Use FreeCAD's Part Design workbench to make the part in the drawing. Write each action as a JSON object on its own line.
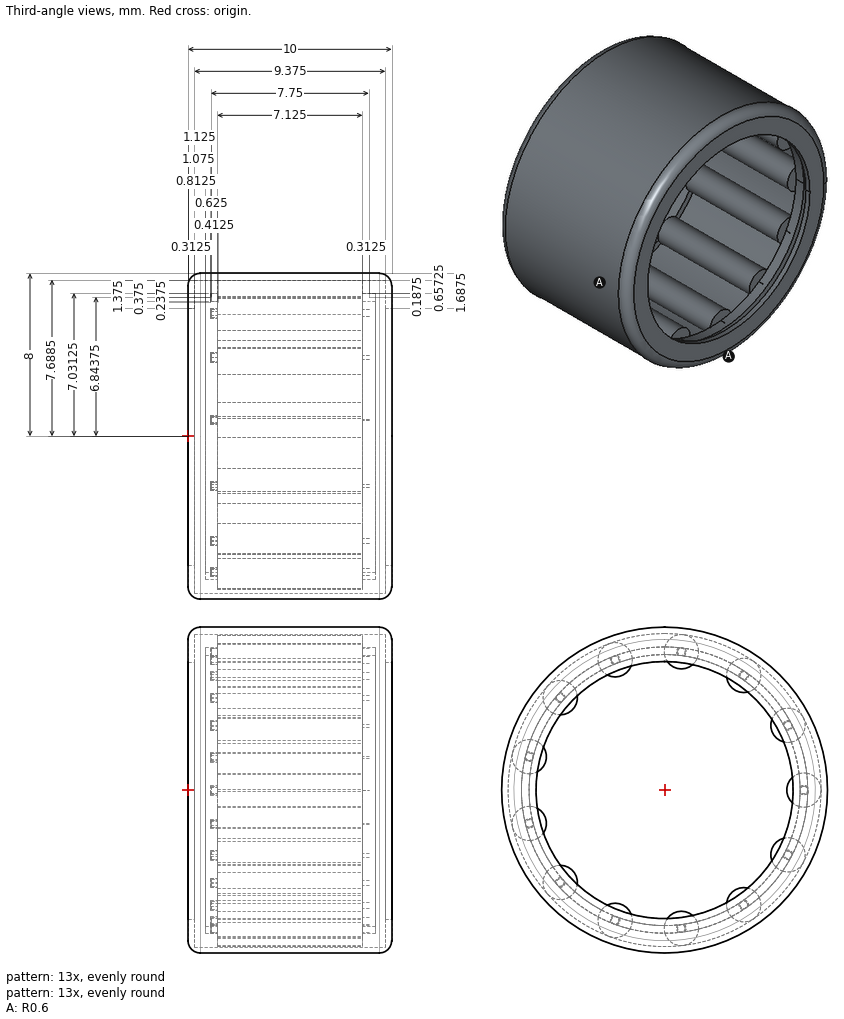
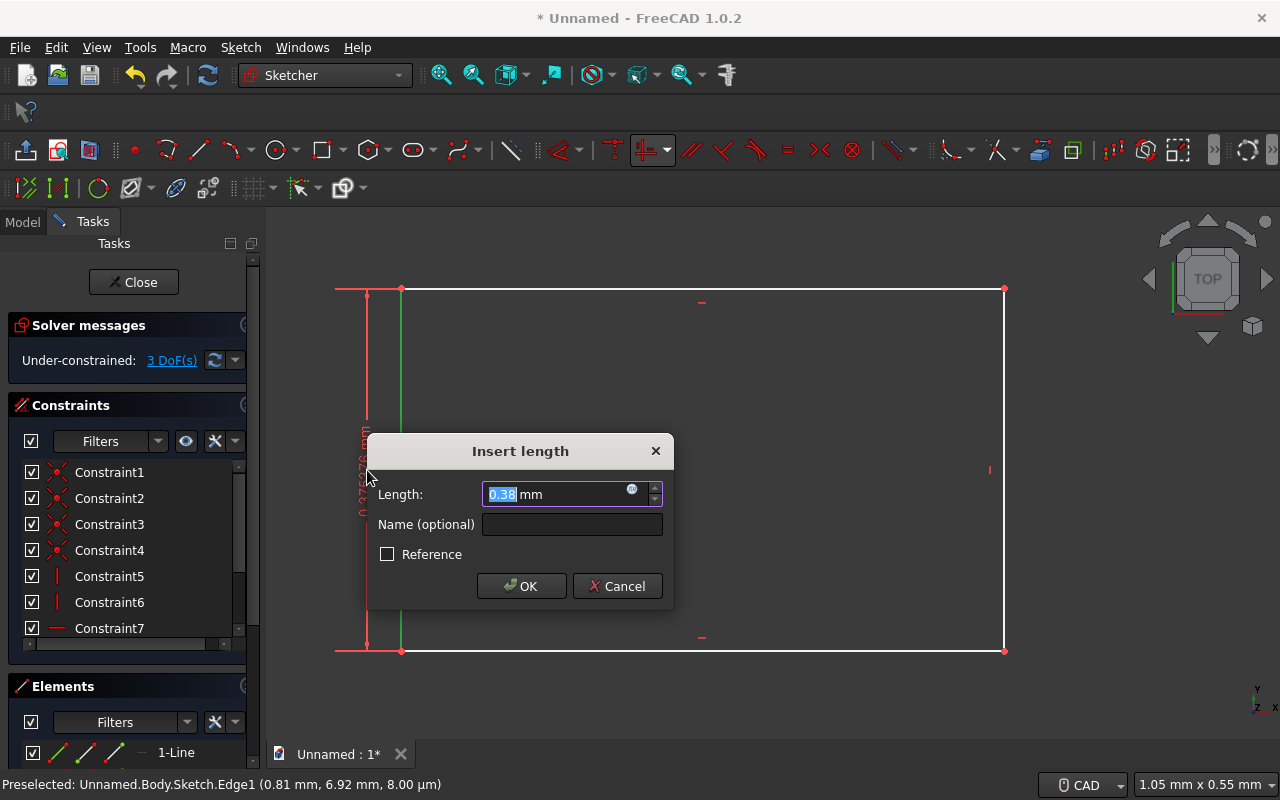
{"action": "type", "text": "0.375"}
{"action": "key", "text": "Return"}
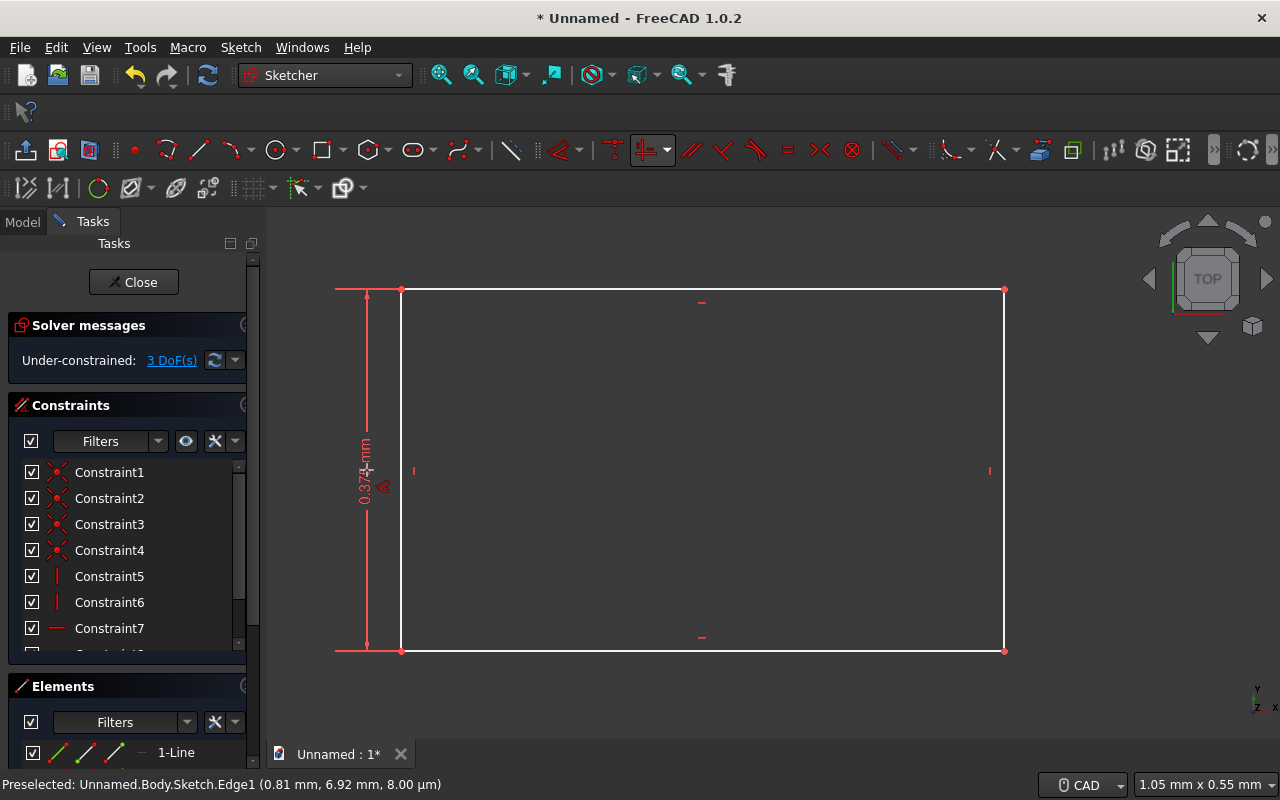
{"action": "left_click", "coordinate": [582, 651]}
{"action": "left_click", "coordinate": [703, 685]}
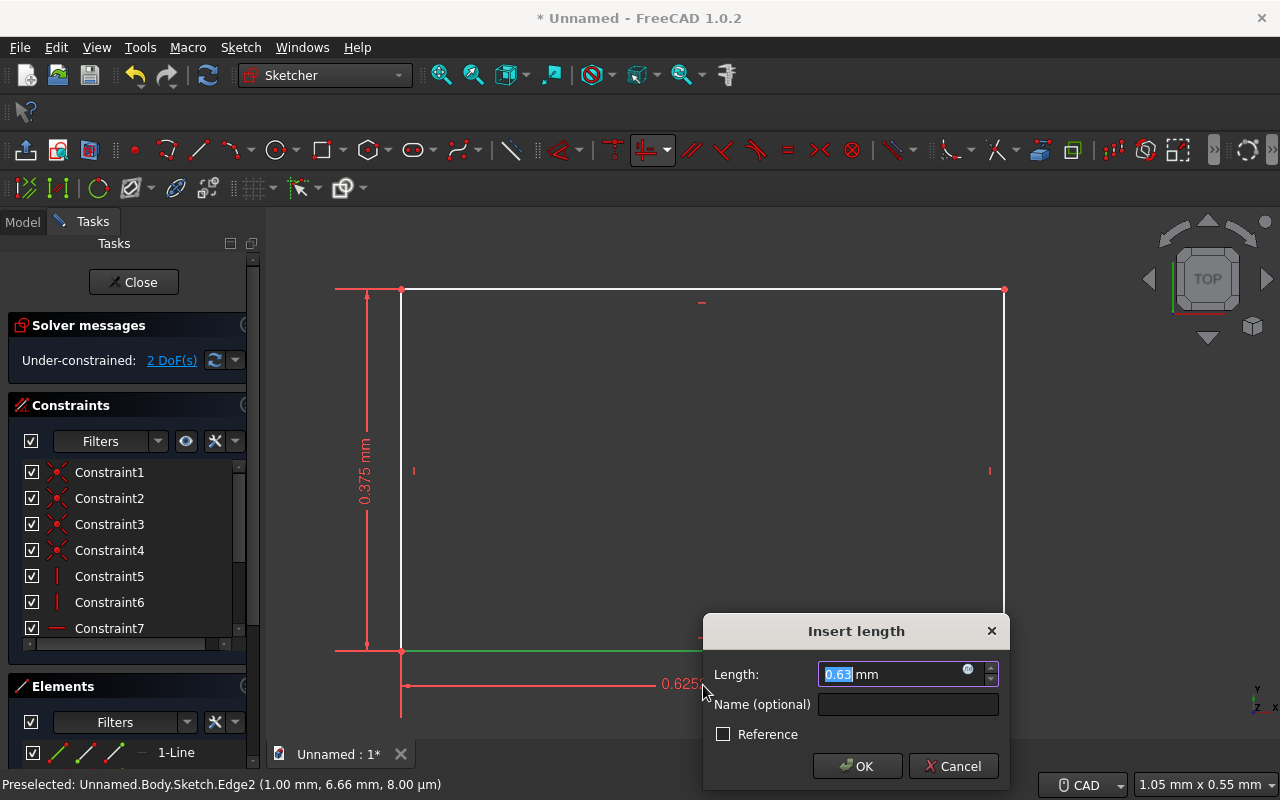
{"action": "type", "text": "0.625"}
{"action": "key", "text": "Return"}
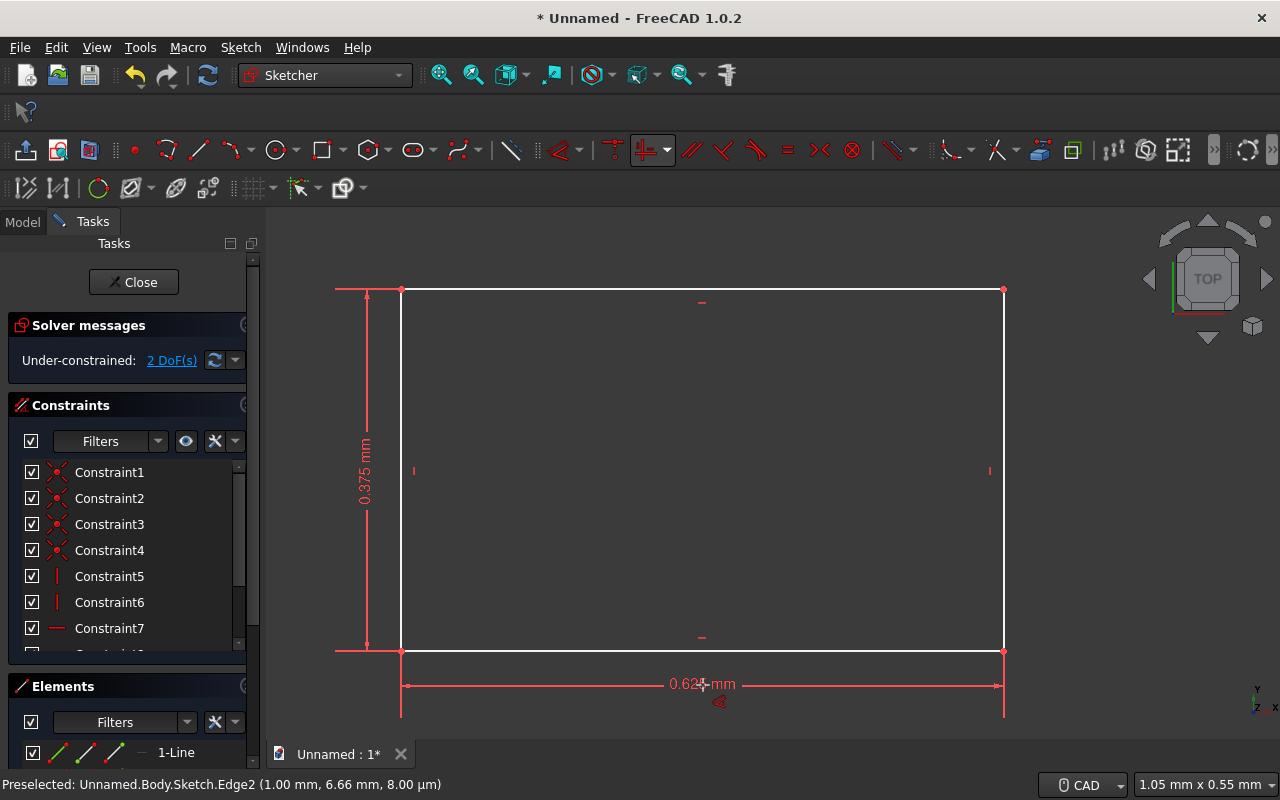
{"action": "left_click", "coordinate": [401, 289]}
{"action": "left_click", "coordinate": [348, 255]}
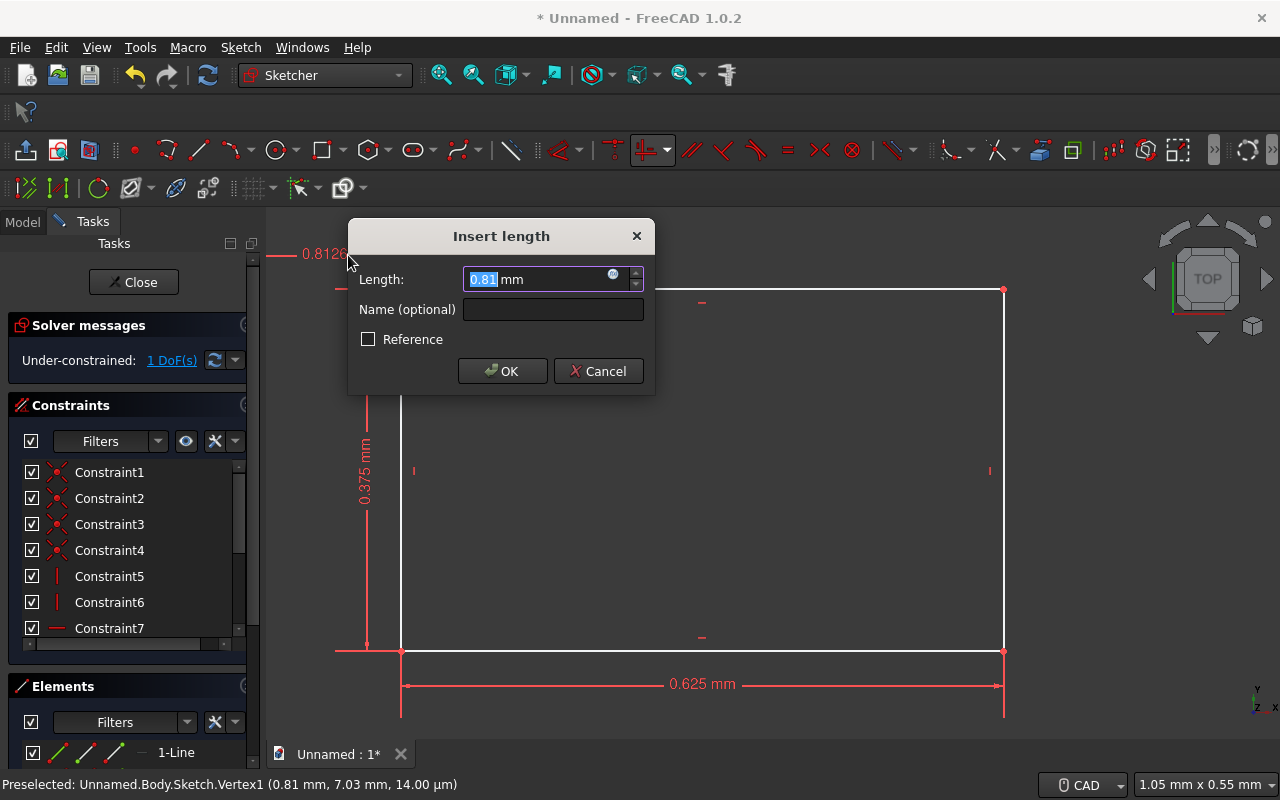
{"action": "type", "text": "0.8125"}
{"action": "key", "text": "Return"}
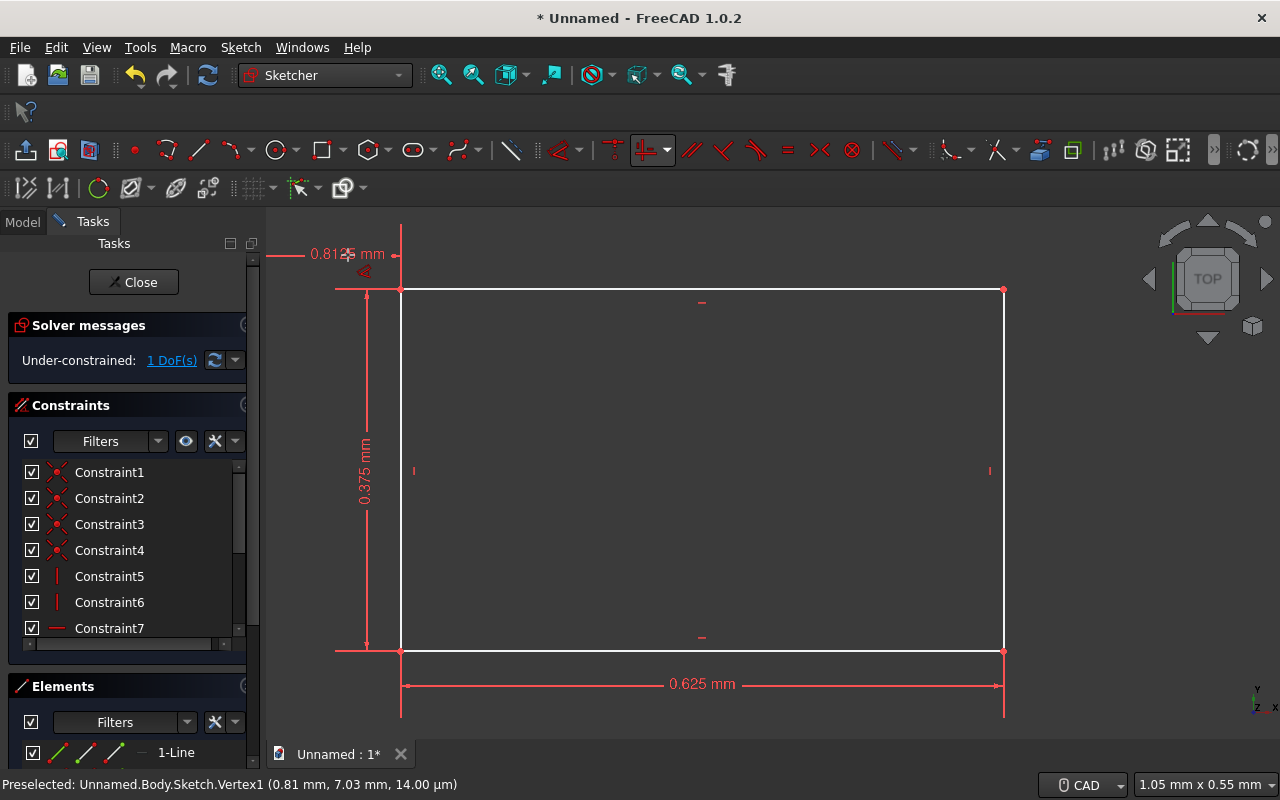
{"action": "left_click", "coordinate": [401, 289]}
{"action": "left_click", "coordinate": [435, 500]}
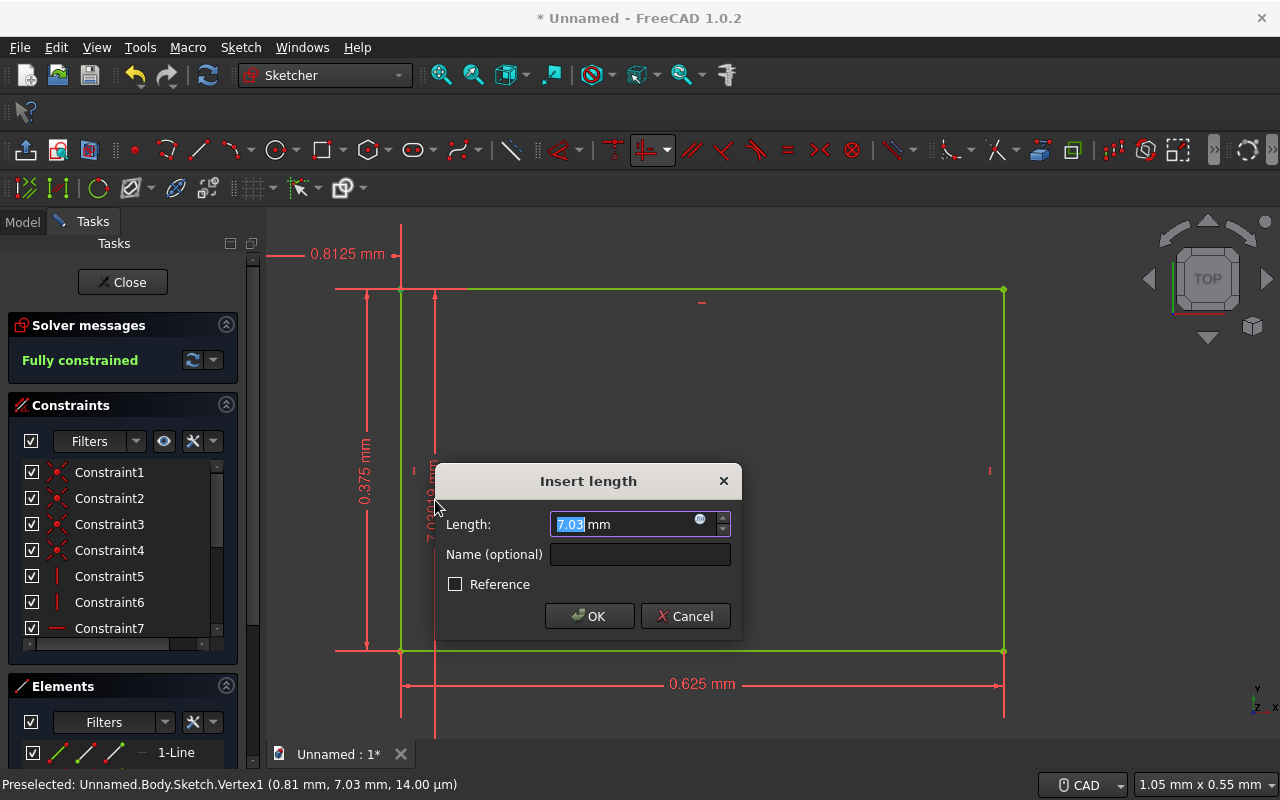
{"action": "type", "text": "7.03125"}
{"action": "key", "text": "Return"}
{"action": "key", "text": "Escape"}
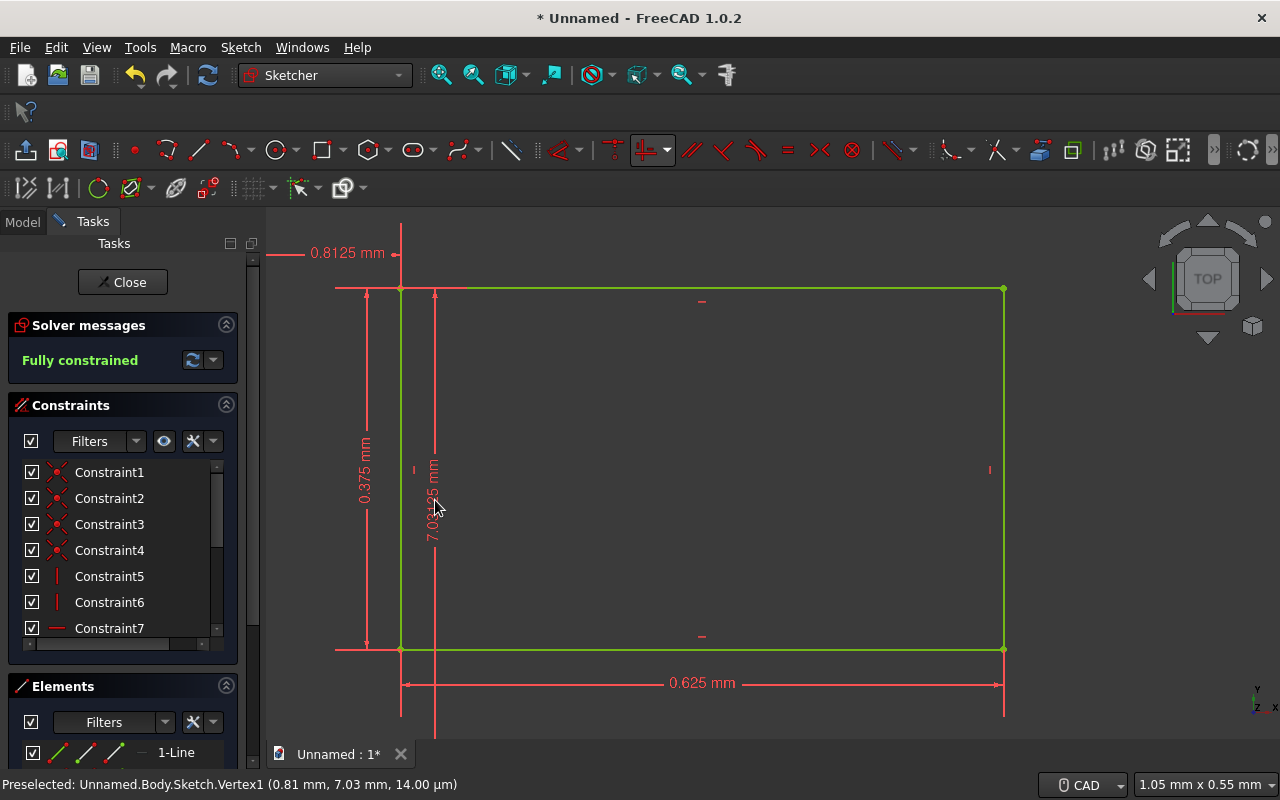
{"action": "left_click", "coordinate": [123, 282]}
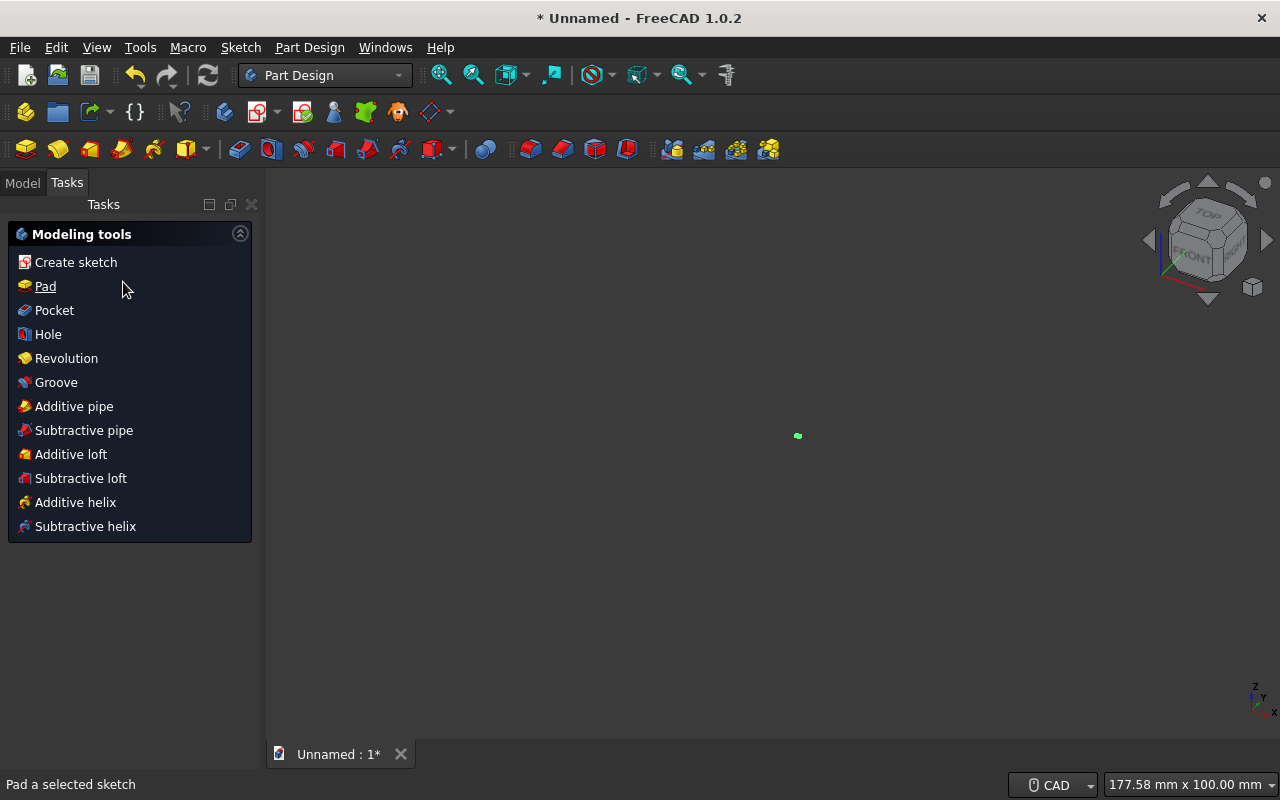
{"action": "left_click", "coordinate": [58, 150]}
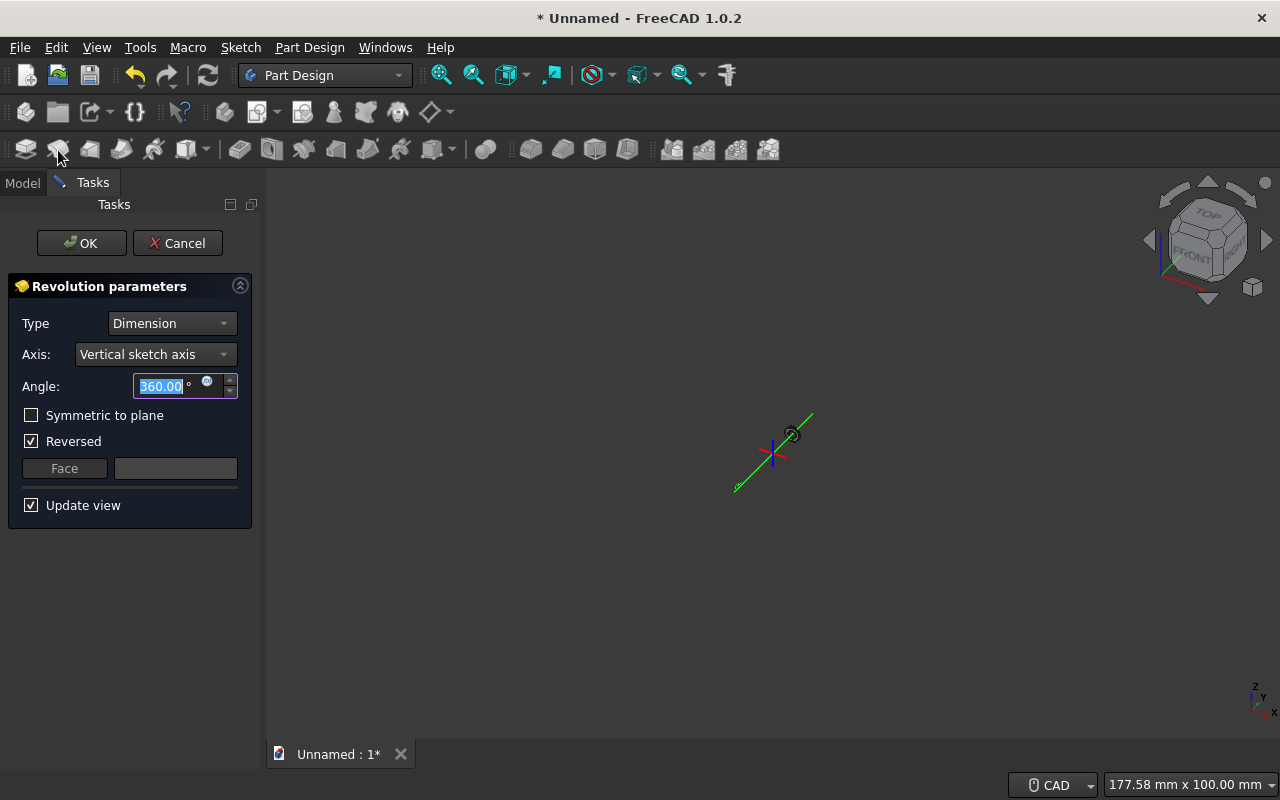
{"action": "left_click", "coordinate": [156, 354]}